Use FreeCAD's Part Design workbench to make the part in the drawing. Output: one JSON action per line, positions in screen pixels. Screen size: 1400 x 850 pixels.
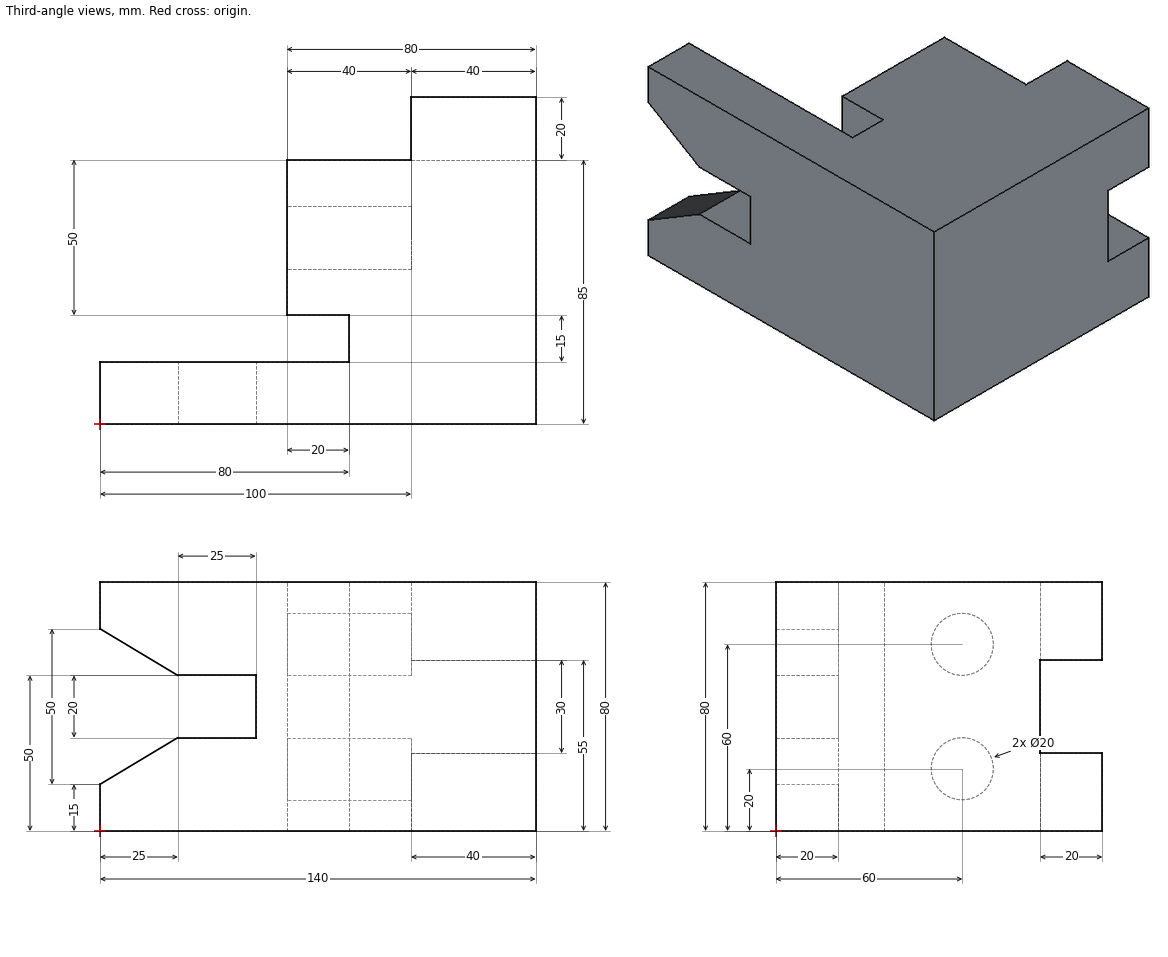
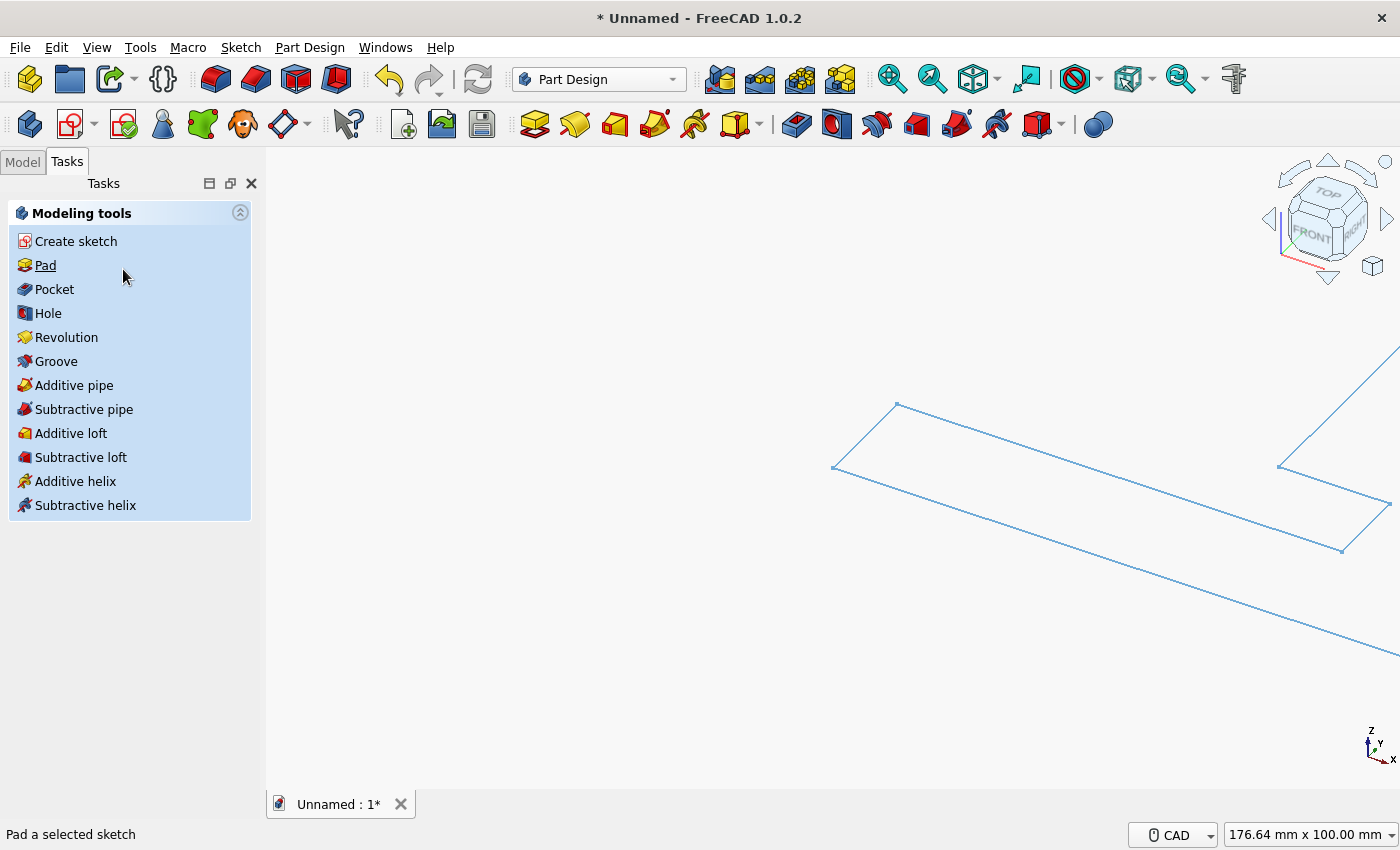
{"action": "left_click", "coordinate": [536, 124]}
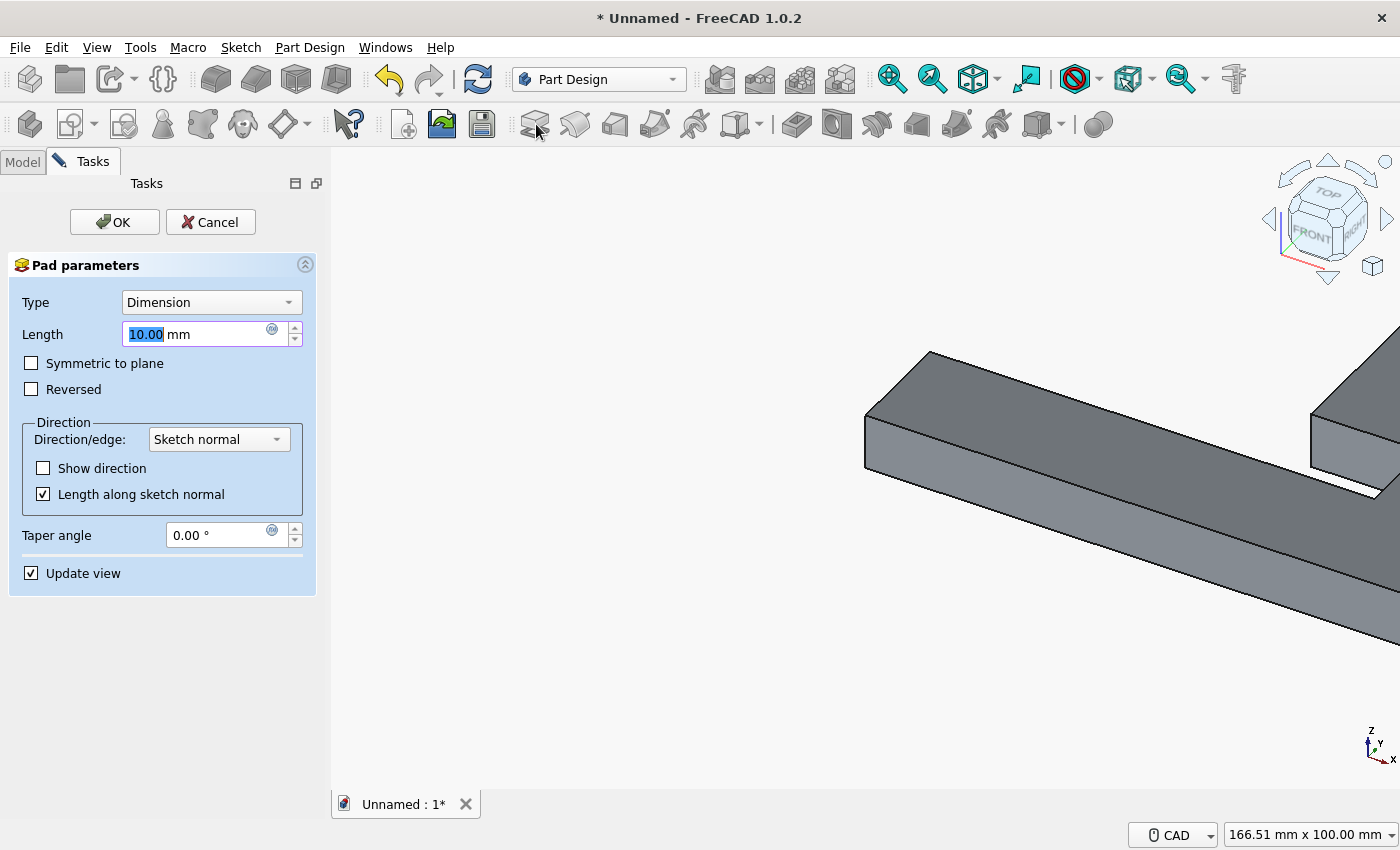
{"action": "type", "text": "80"}
{"action": "key", "text": "Tab"}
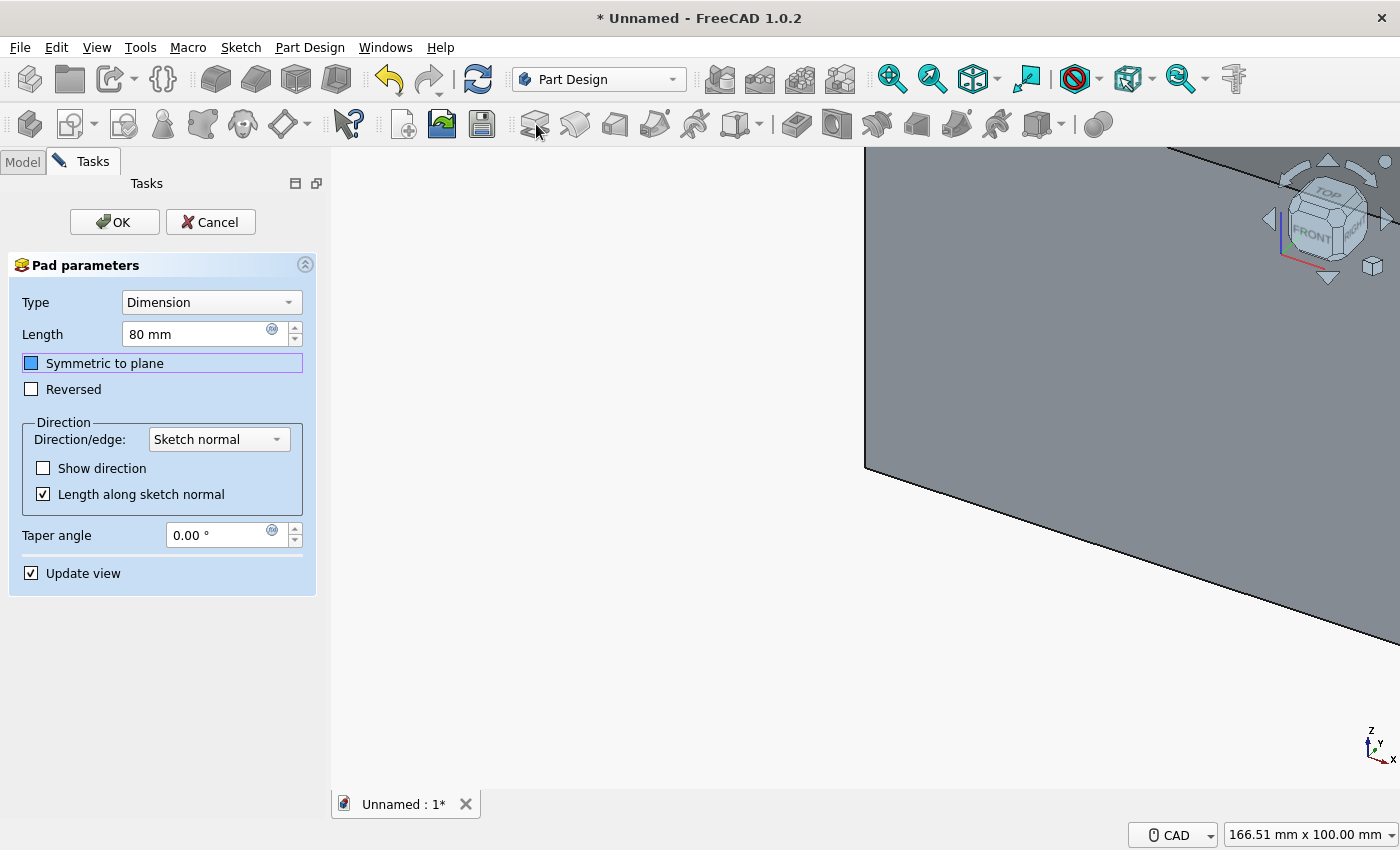
{"action": "left_click", "coordinate": [115, 222]}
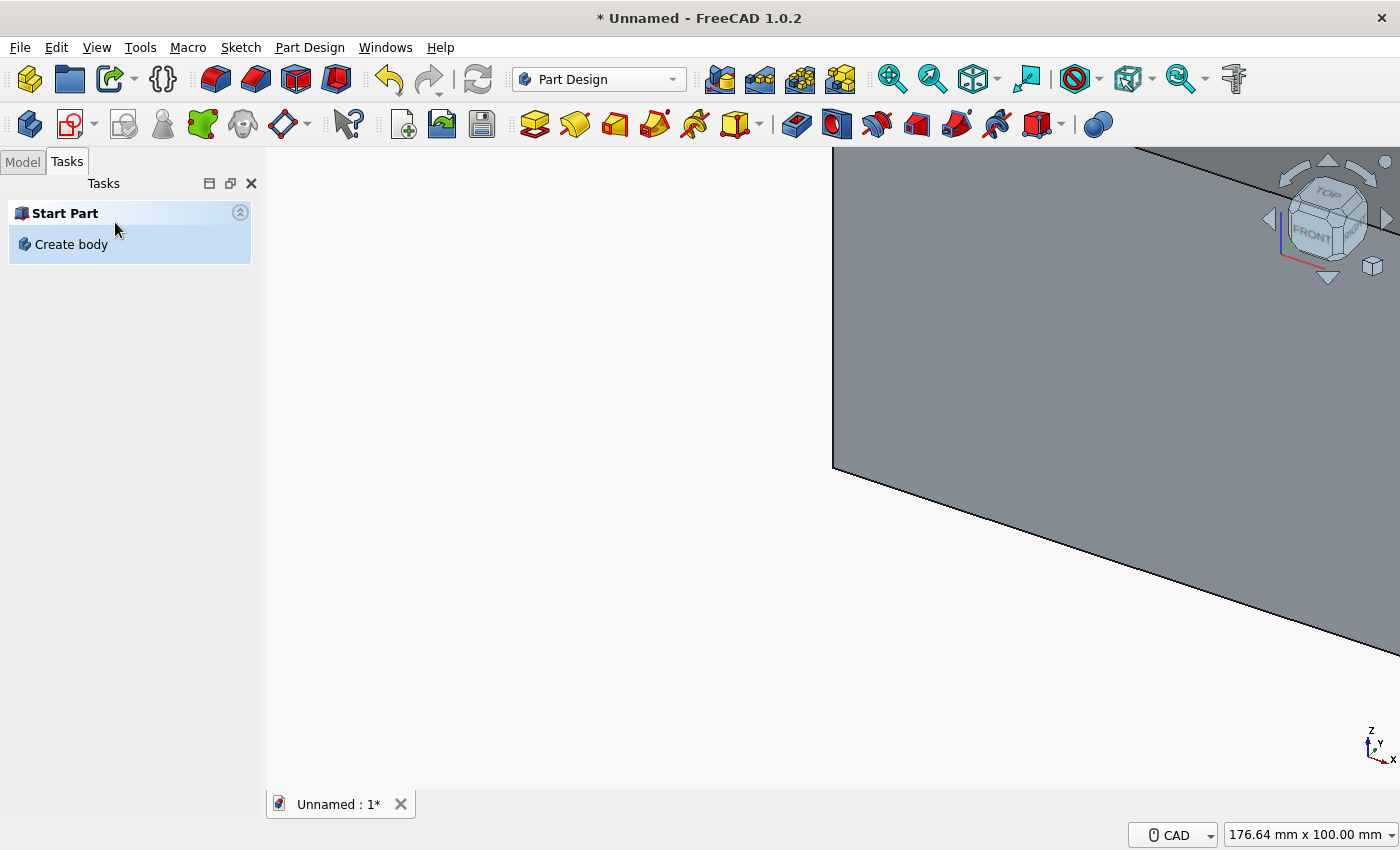
{"action": "key", "text": "v f"}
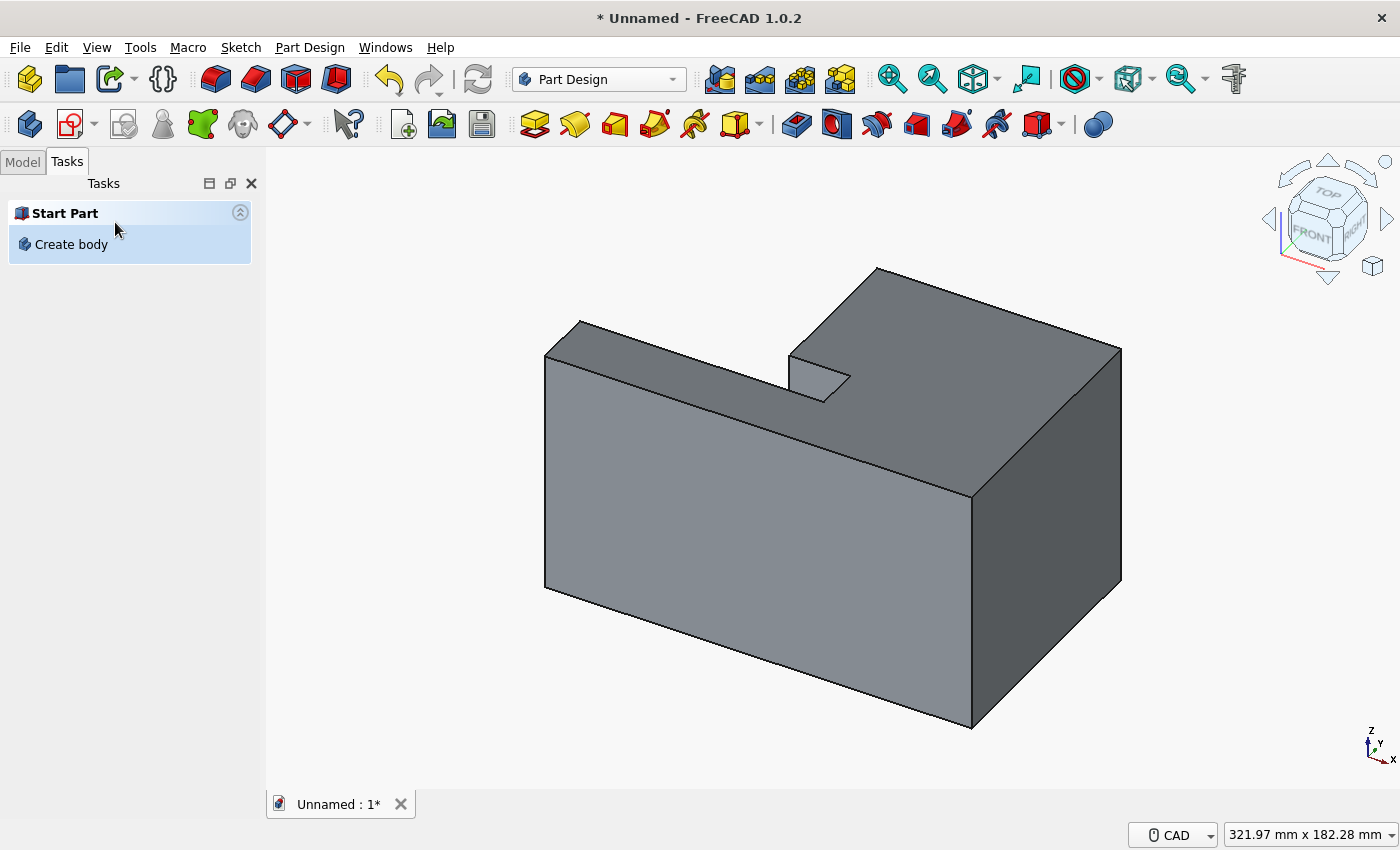
{"action": "left_click", "coordinate": [976, 371]}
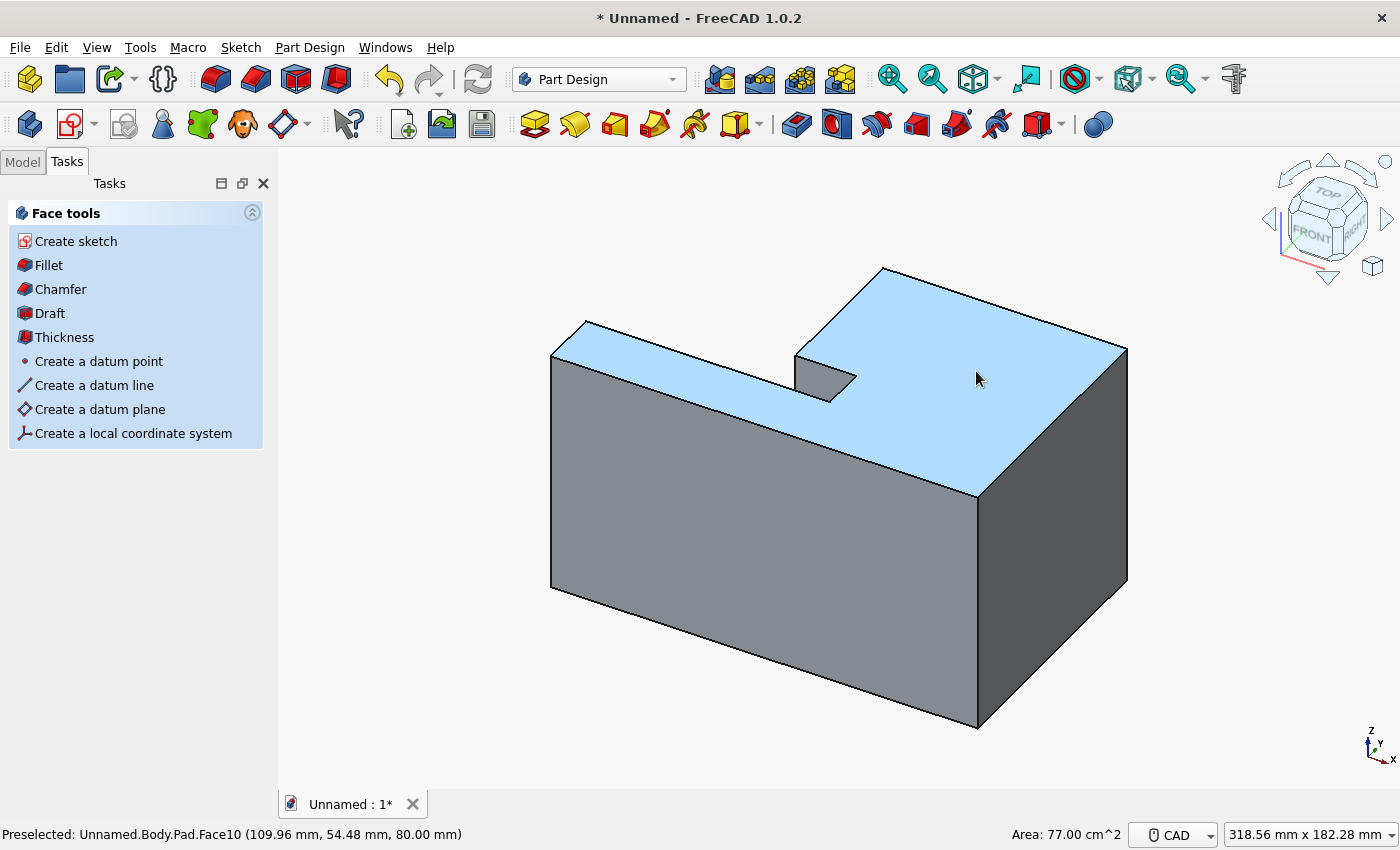
{"action": "left_click", "coordinate": [70, 124]}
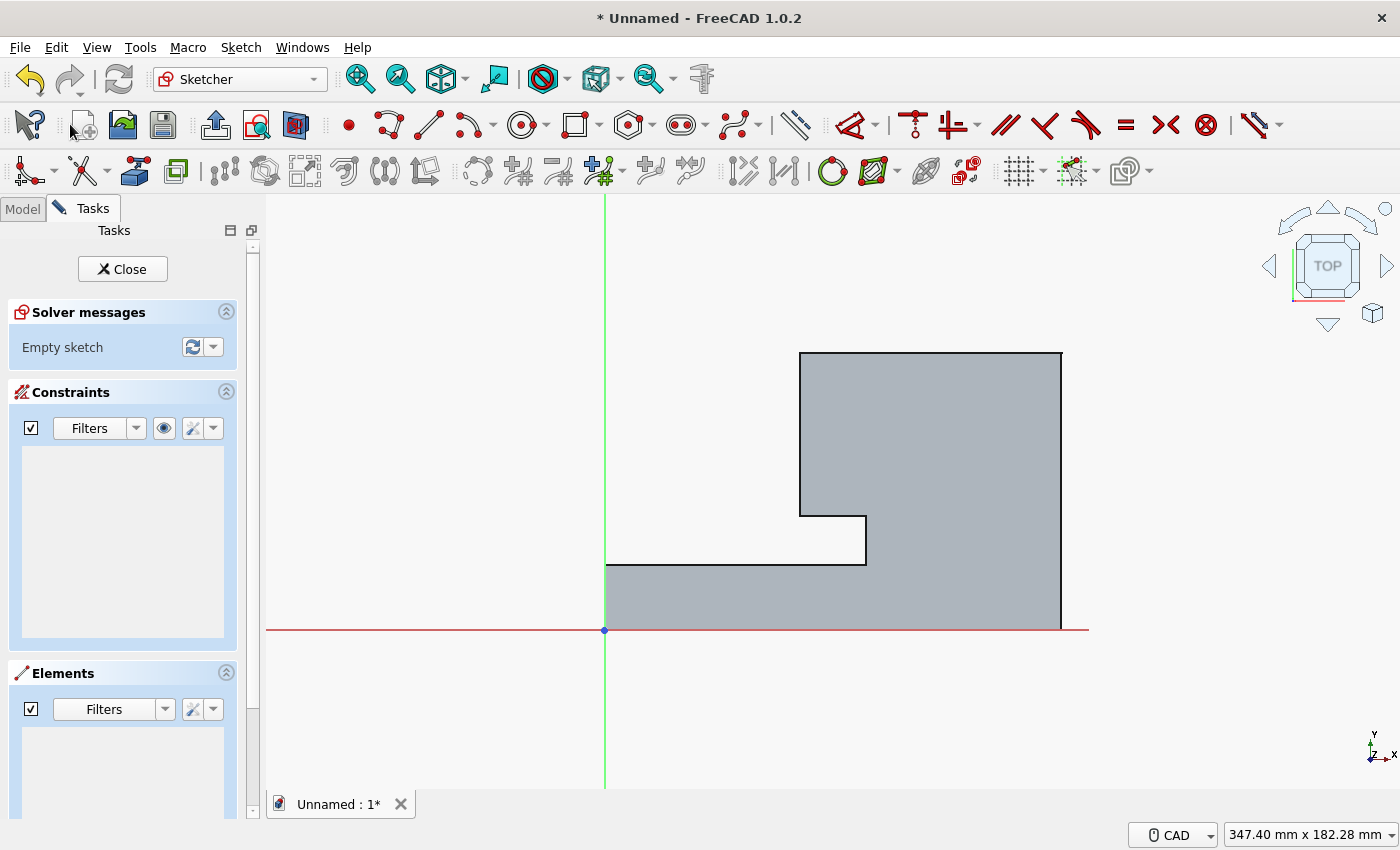
{"action": "scroll", "coordinate": [1055, 277], "scroll_direction": "up", "scroll_amount": 8}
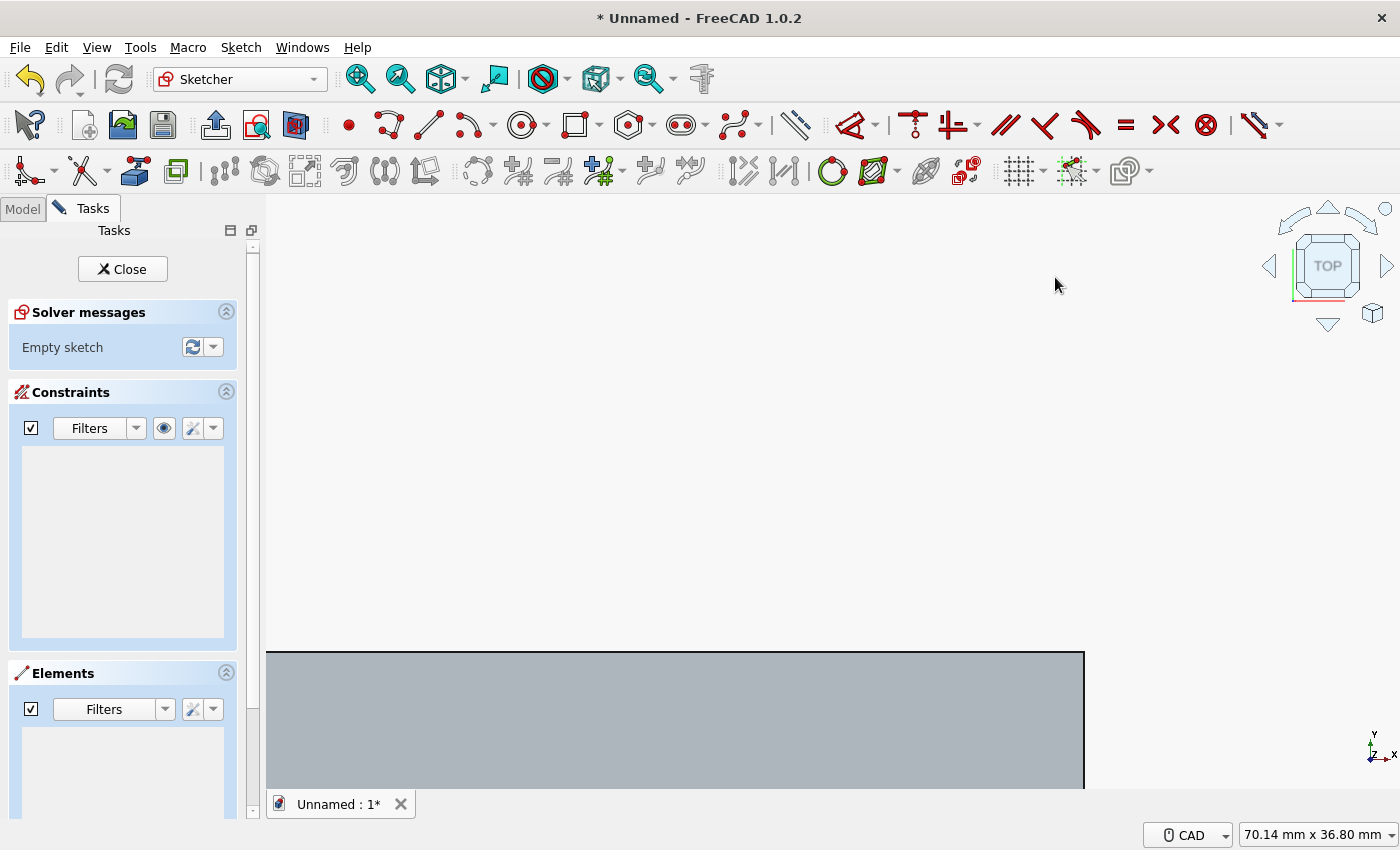
{"action": "key", "text": "g r"}